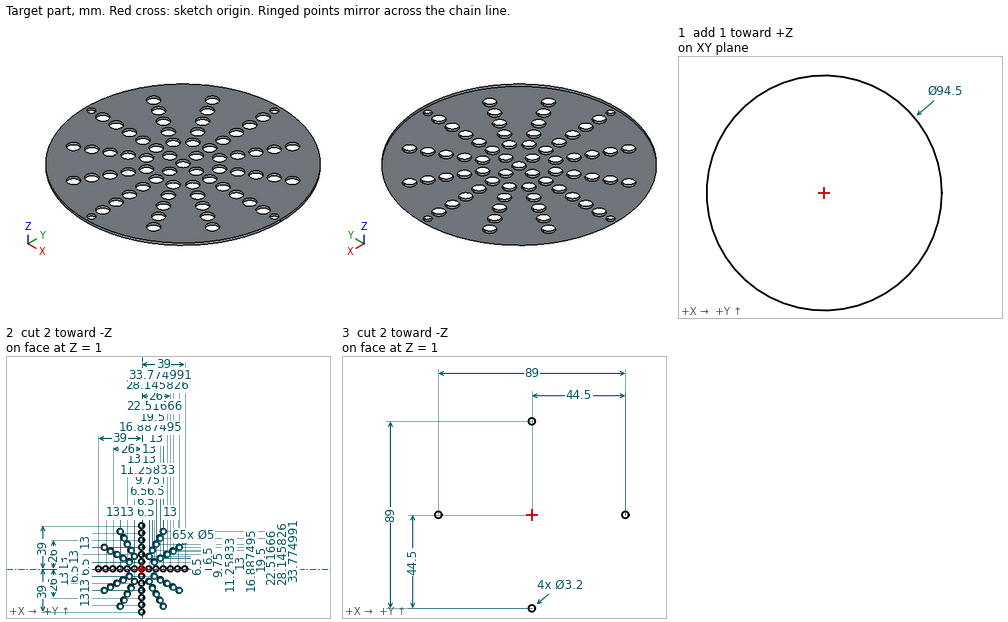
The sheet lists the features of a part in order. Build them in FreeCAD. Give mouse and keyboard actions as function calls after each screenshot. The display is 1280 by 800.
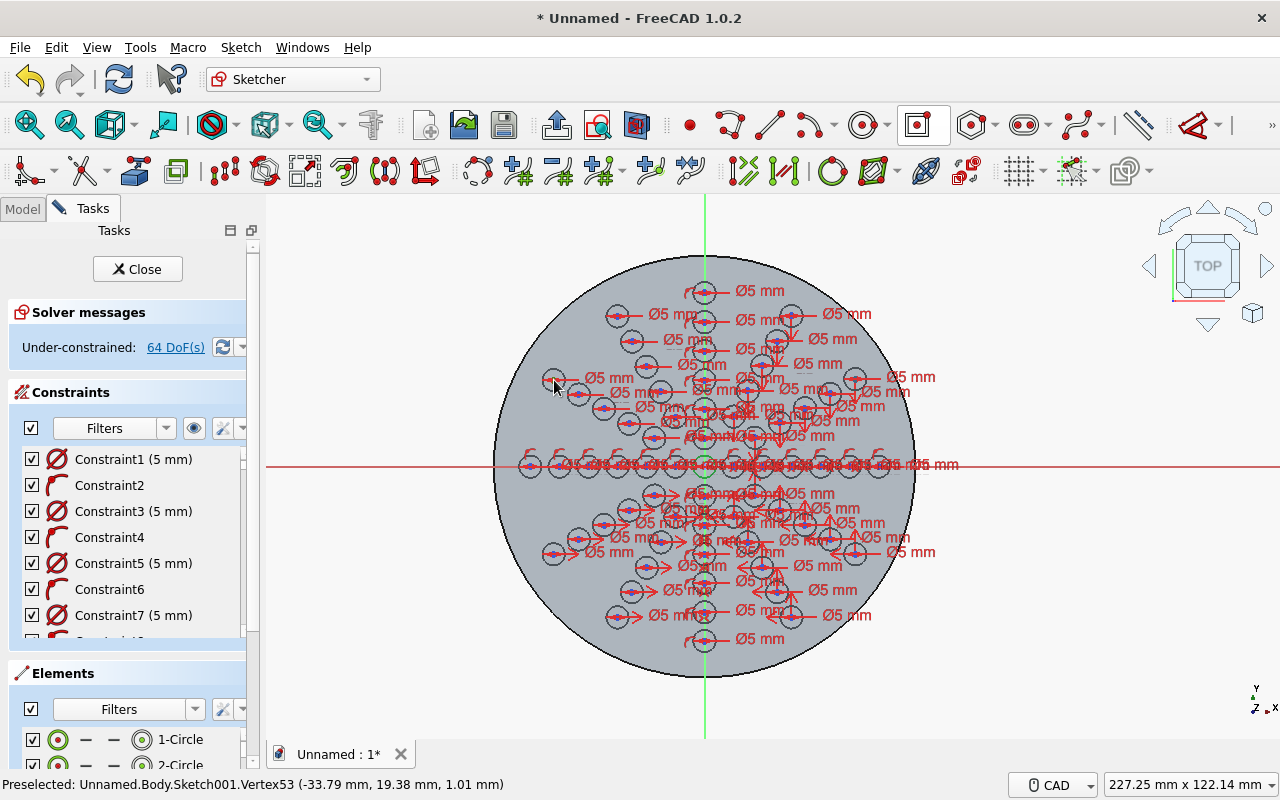
click(705, 257)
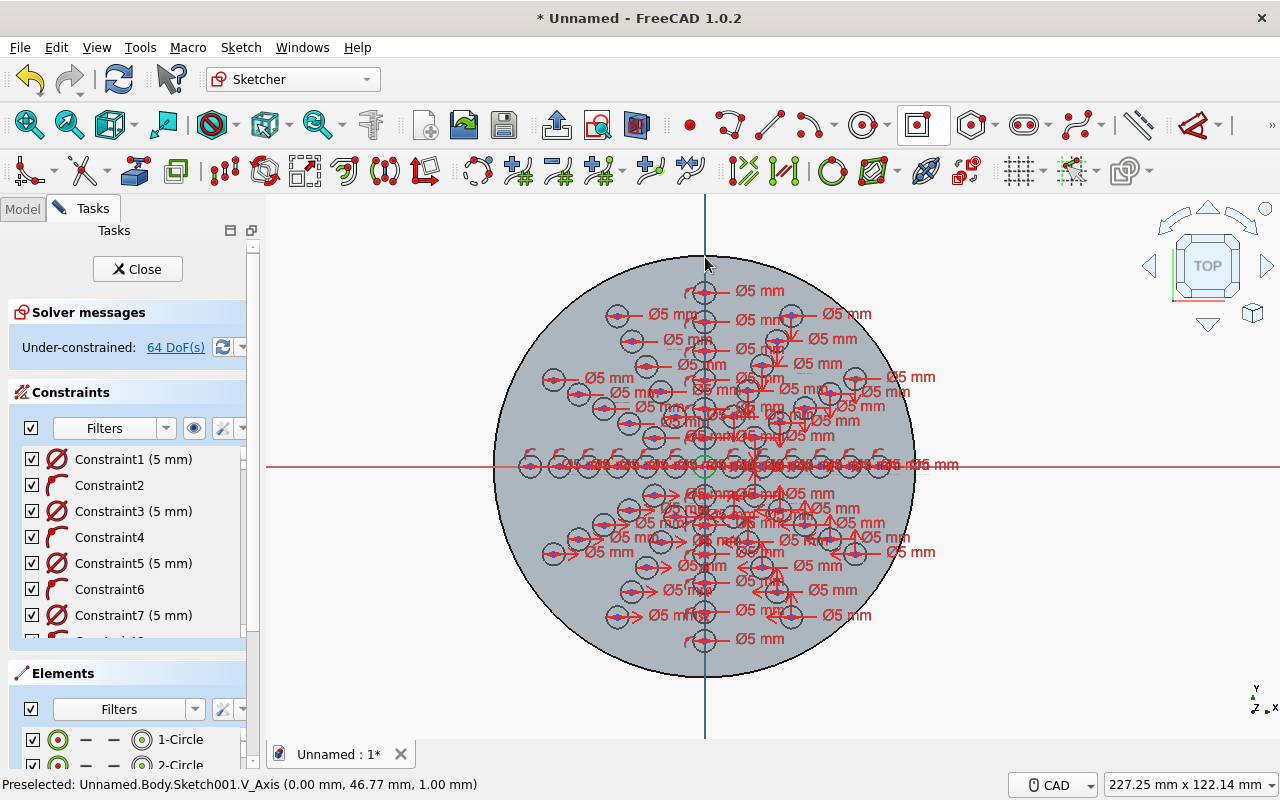
key(s)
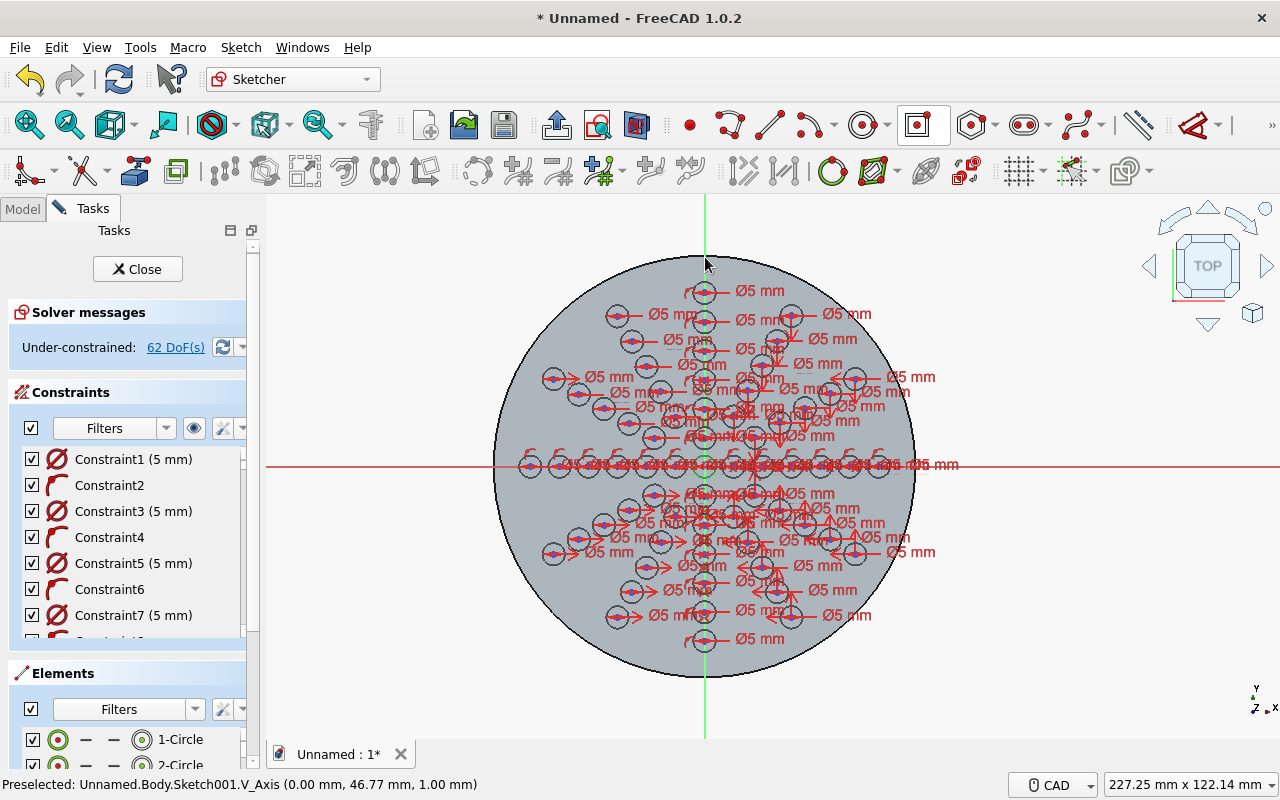
click(830, 394)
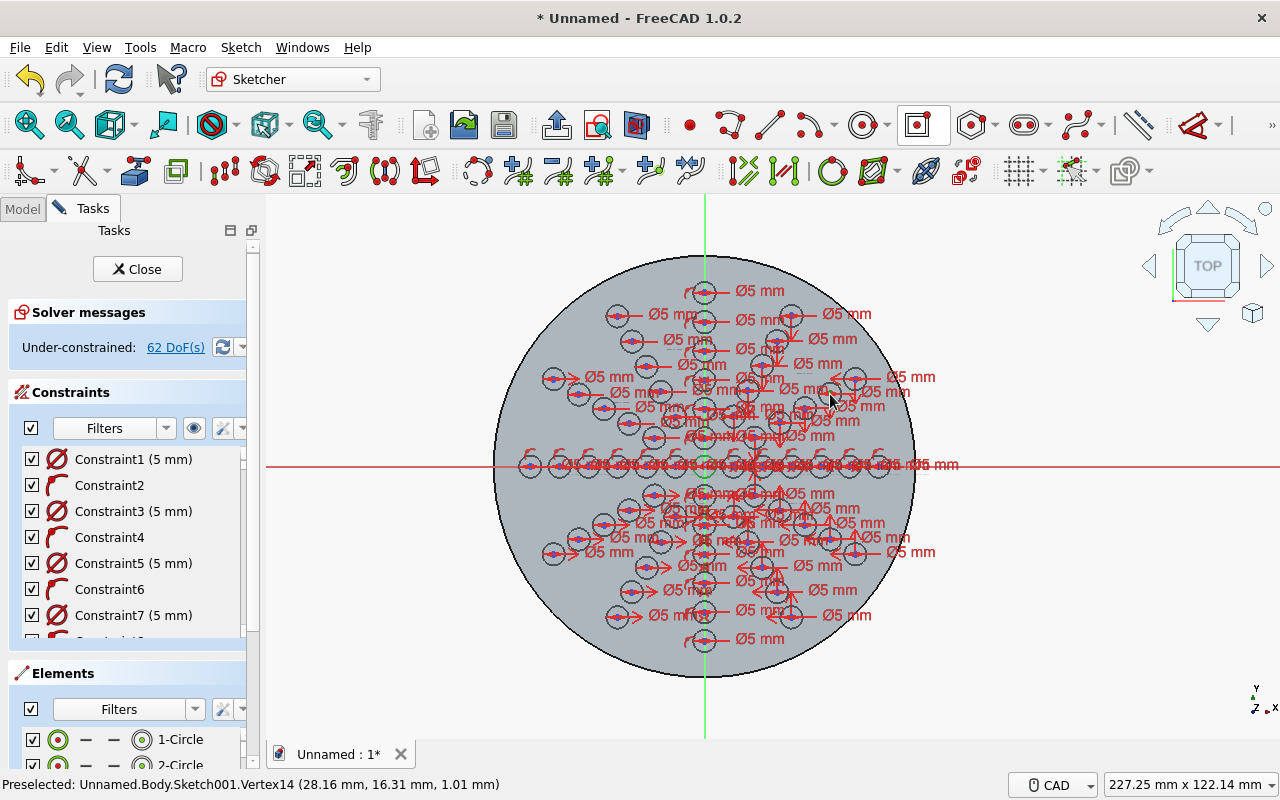
click(579, 395)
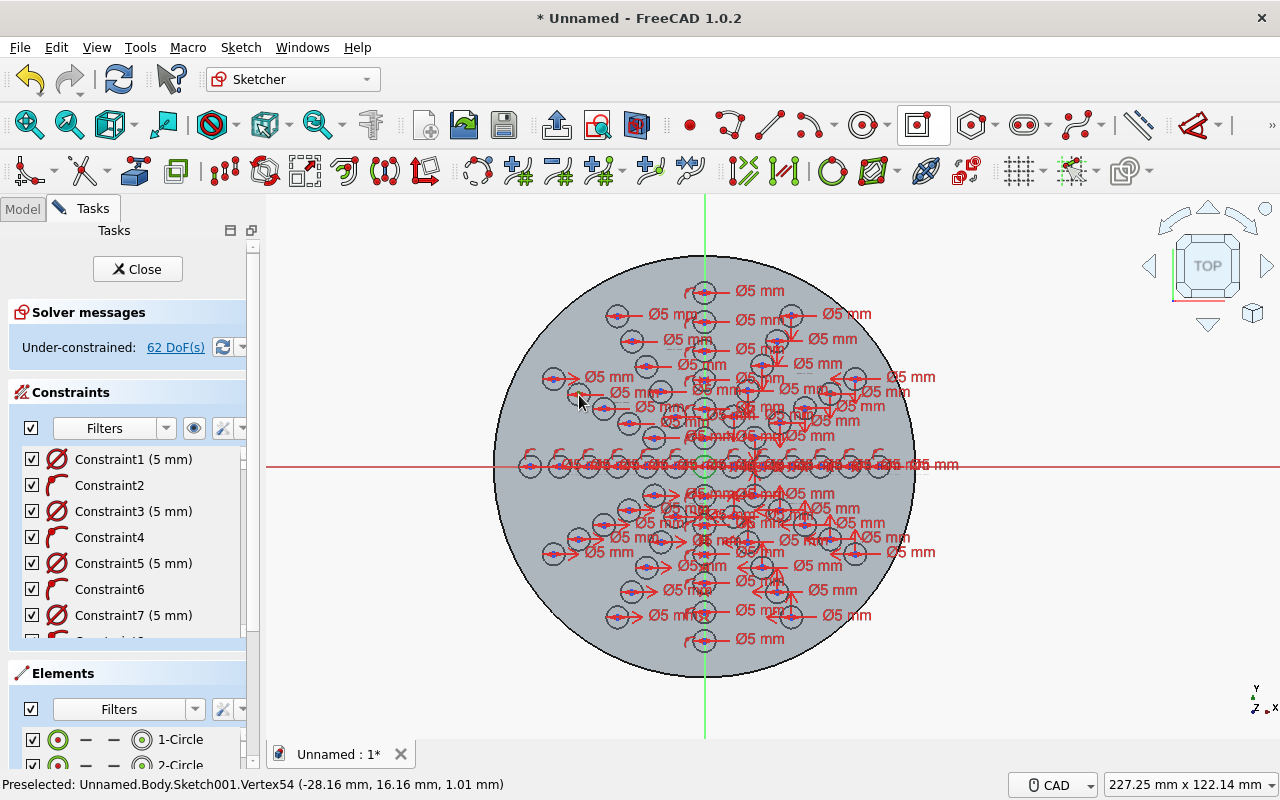
click(705, 257)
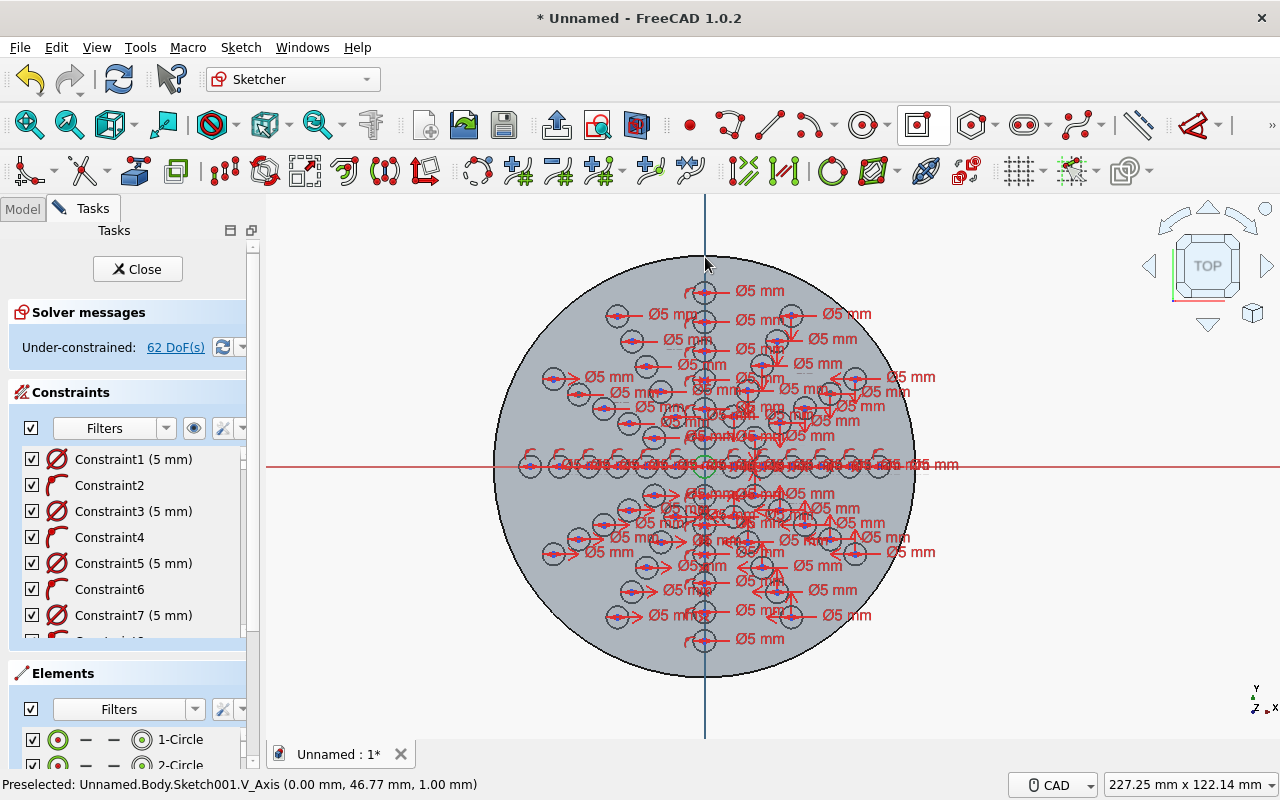
key(s)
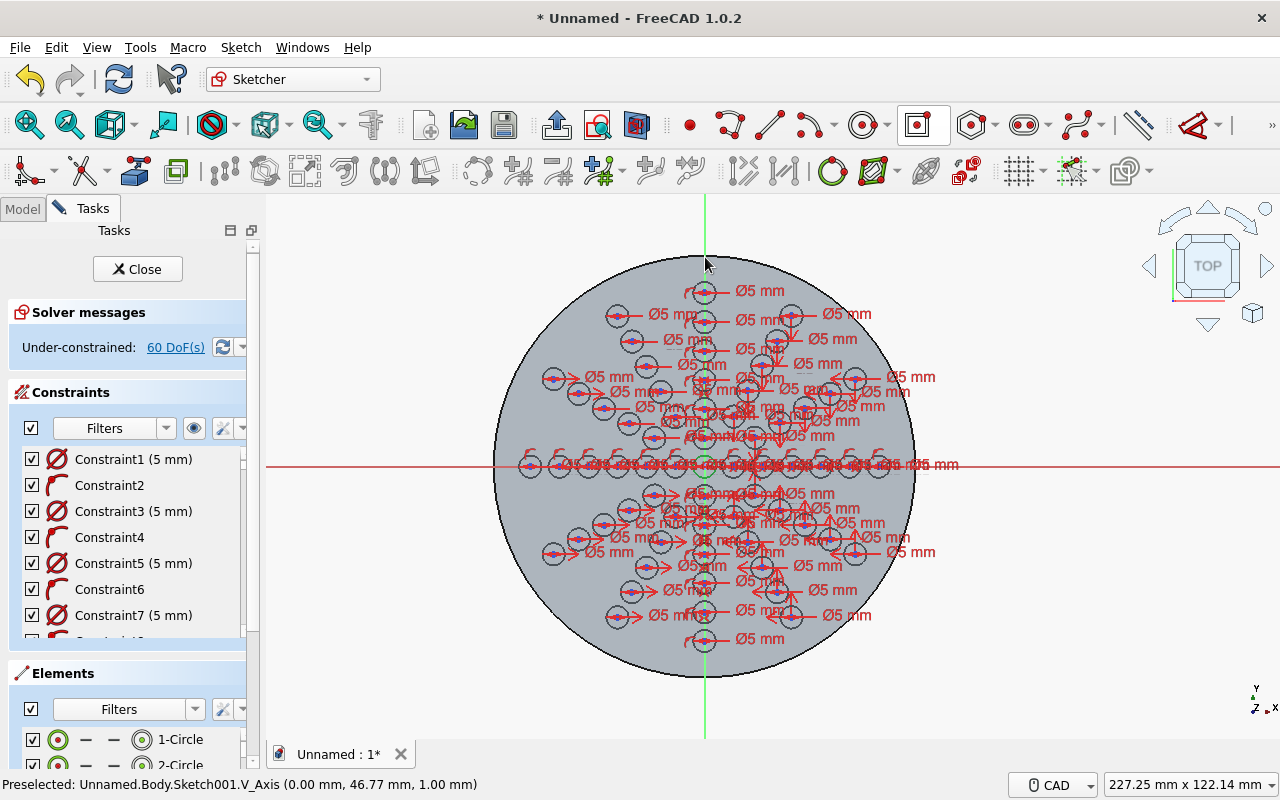
click(805, 408)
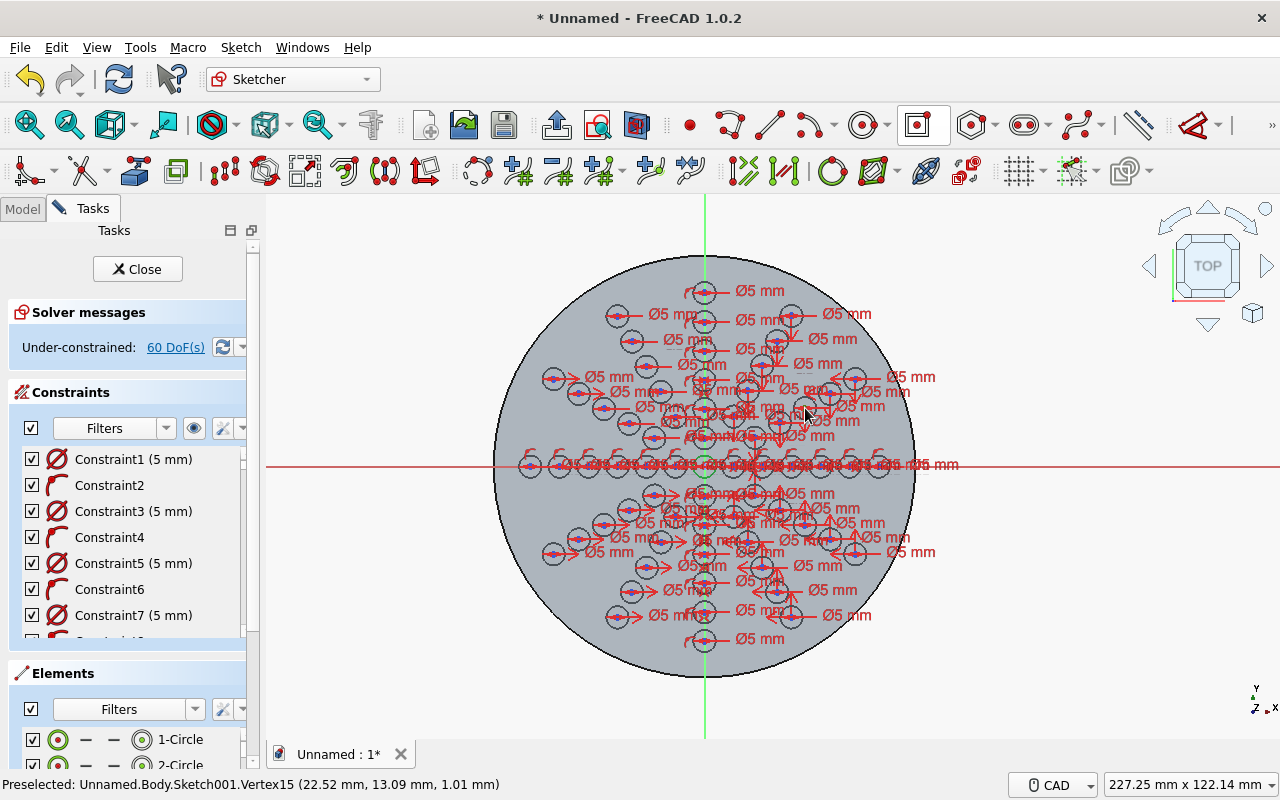
click(604, 409)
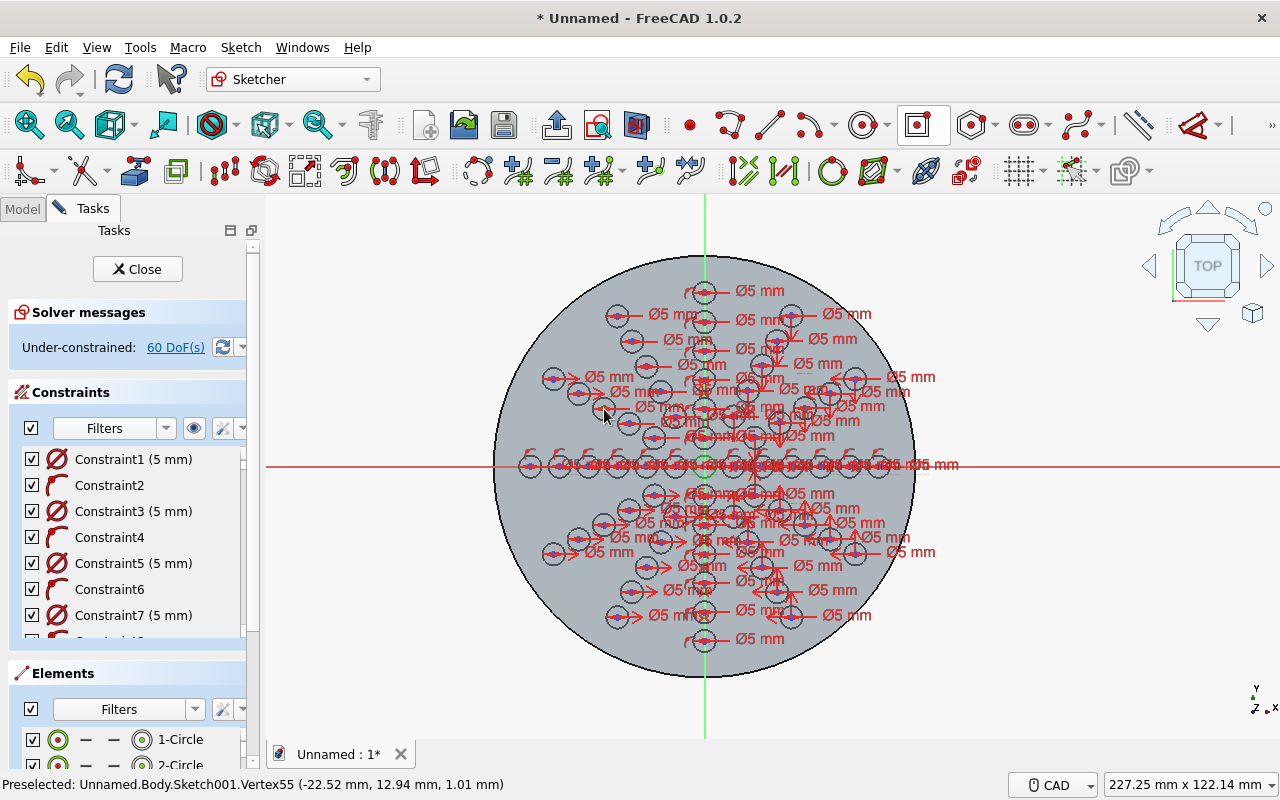
click(705, 257)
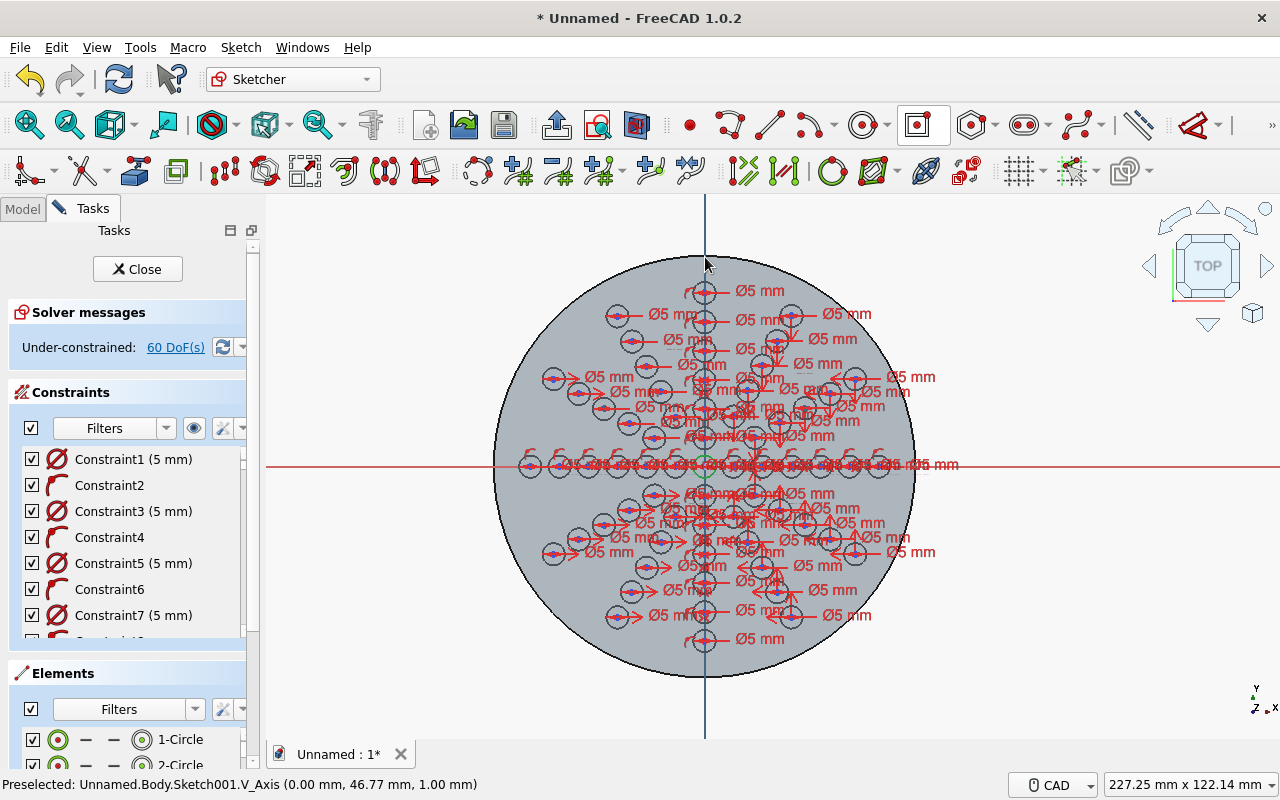
key(s)